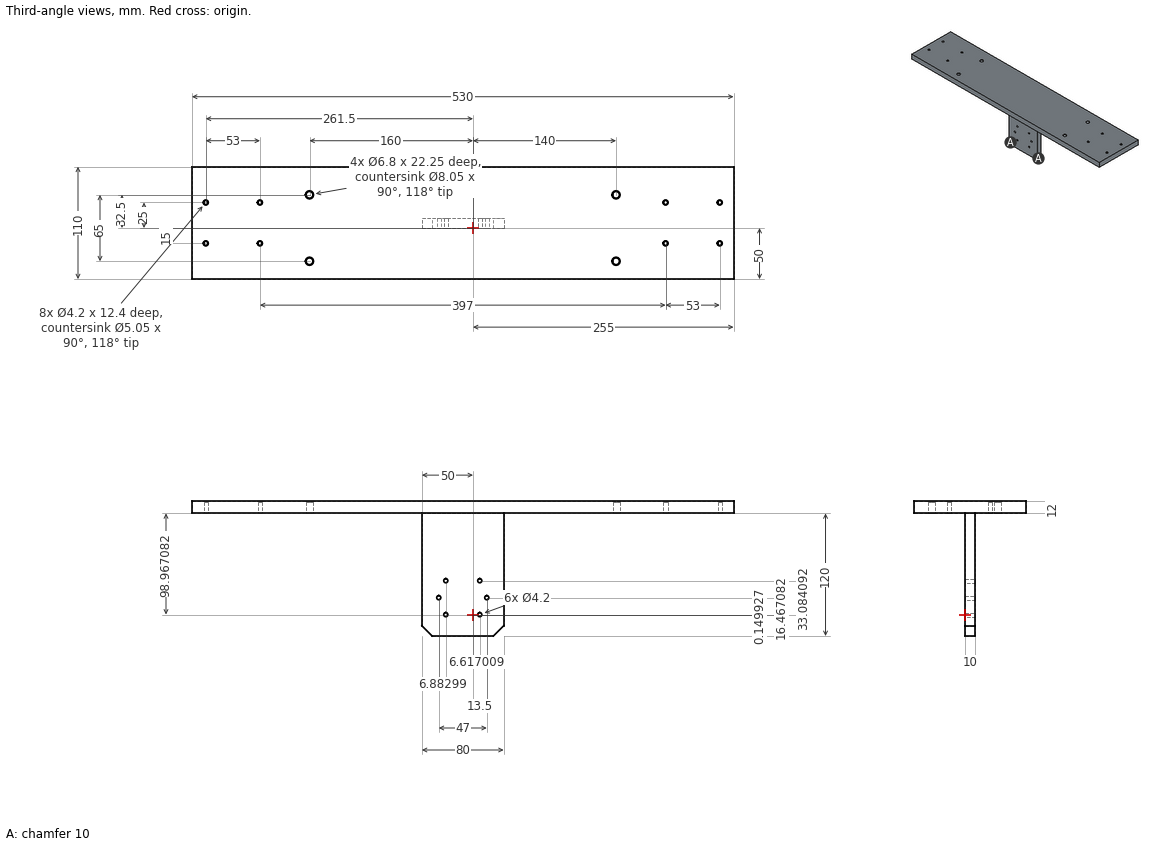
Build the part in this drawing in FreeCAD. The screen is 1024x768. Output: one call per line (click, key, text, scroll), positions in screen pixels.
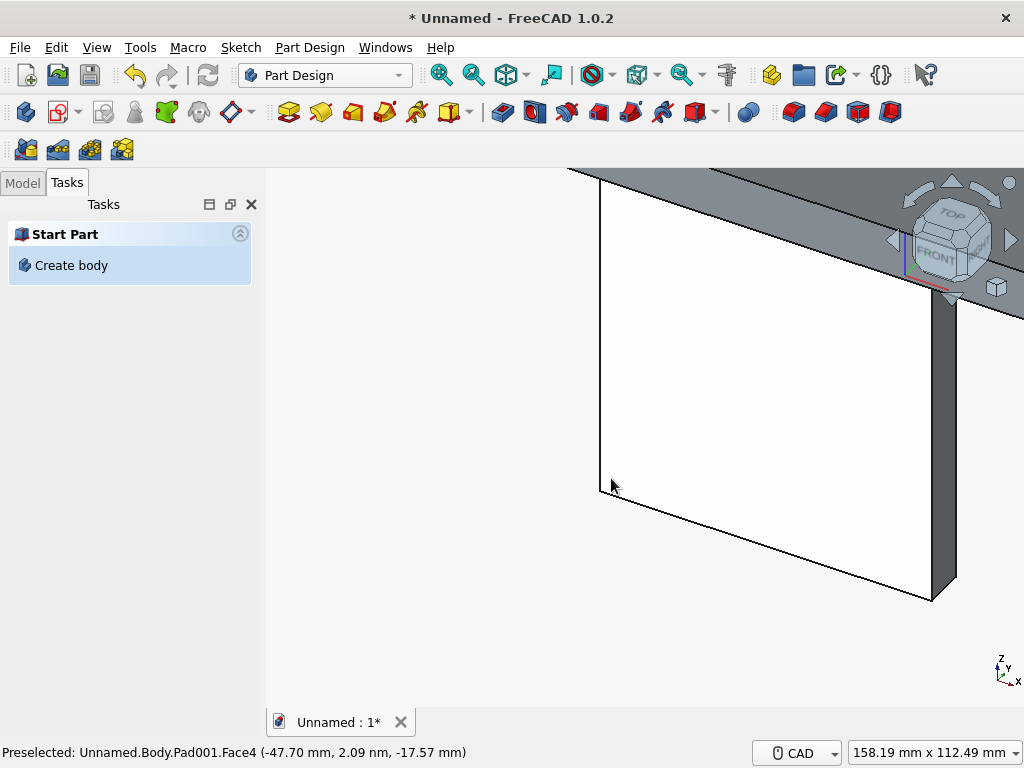
click(442, 76)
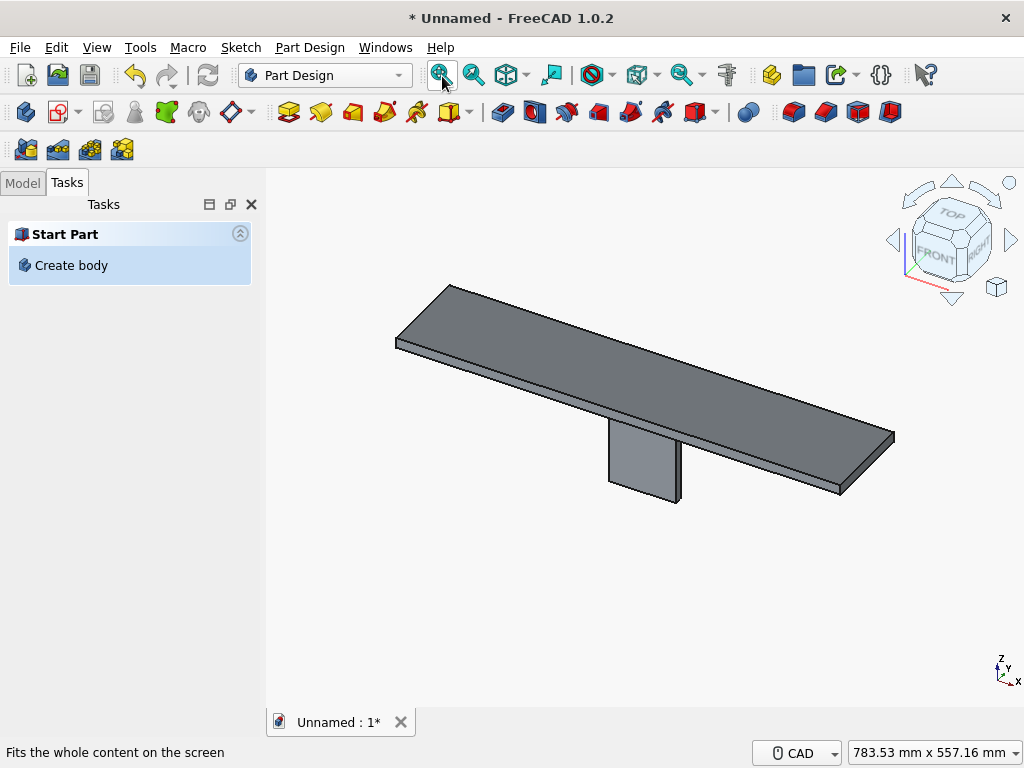
key(0)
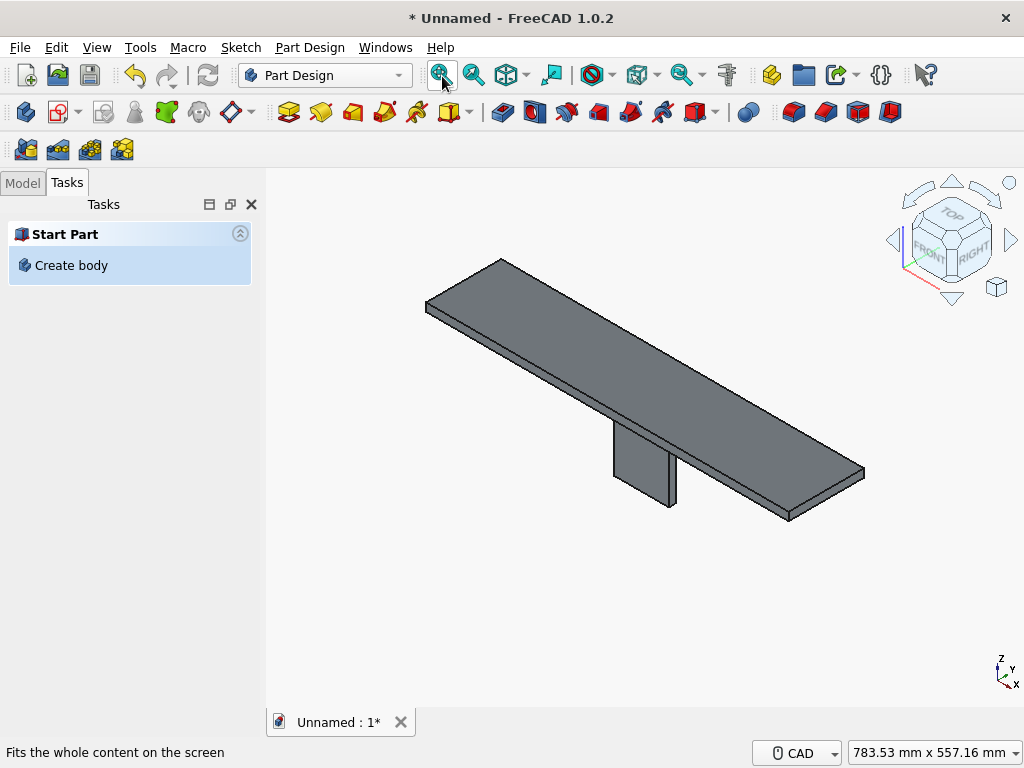
scroll(618, 473, up, 8)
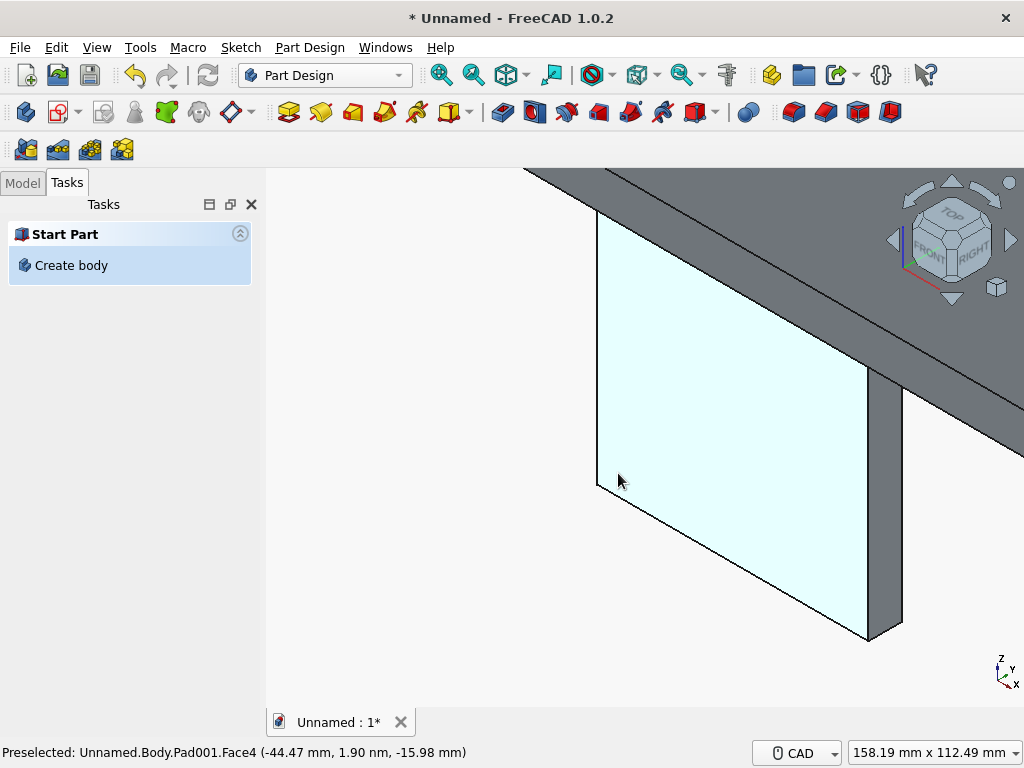
key(v)
key(f)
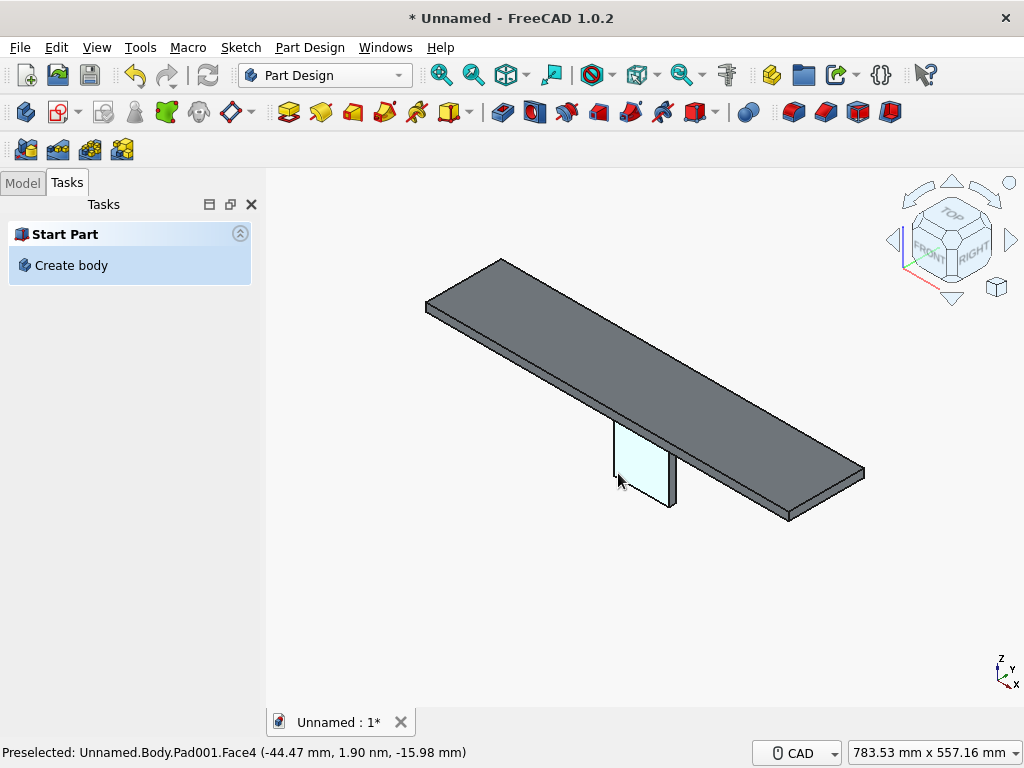
key(2)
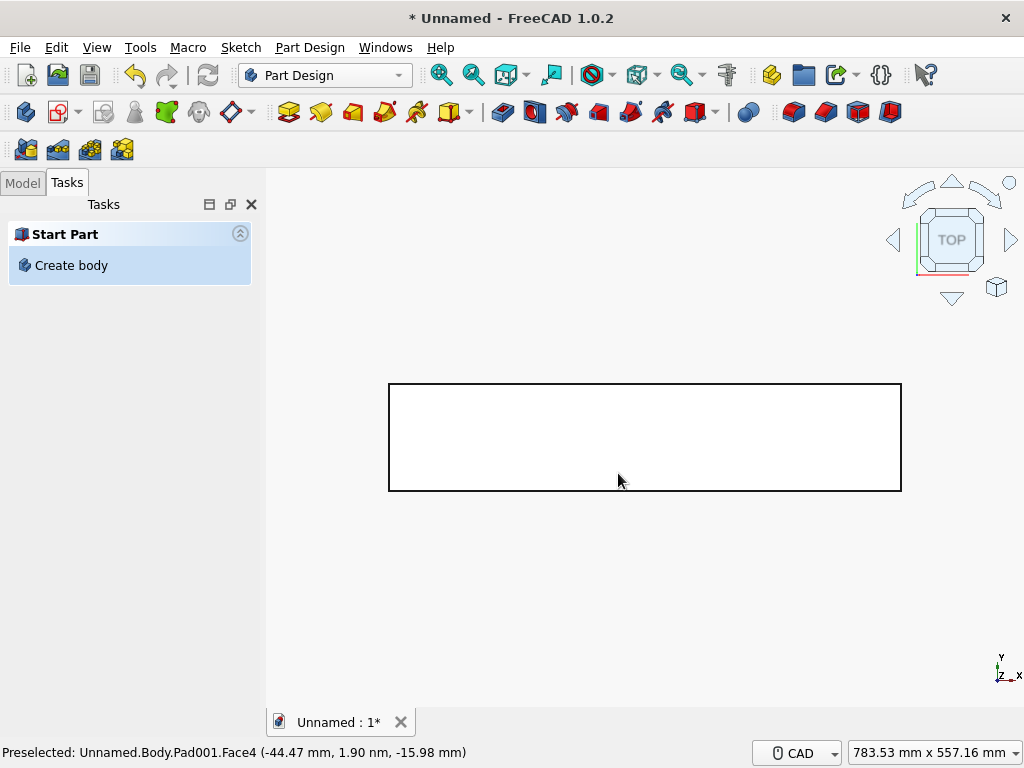
scroll(606, 436, up, 8)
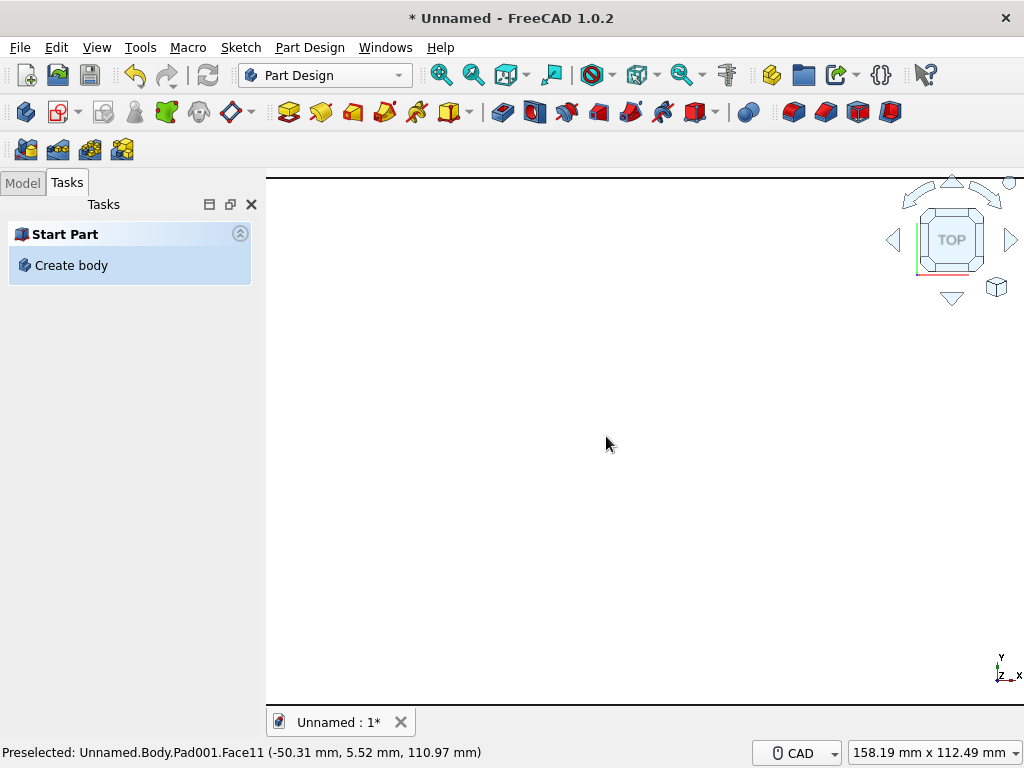
click(442, 76)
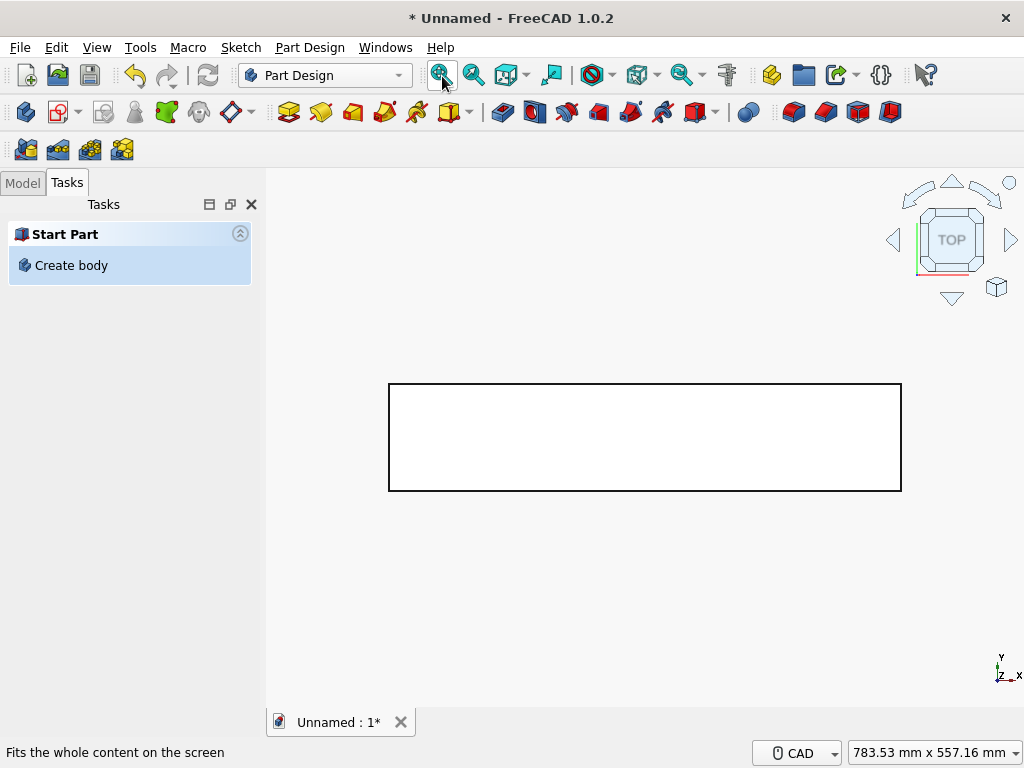
key(1)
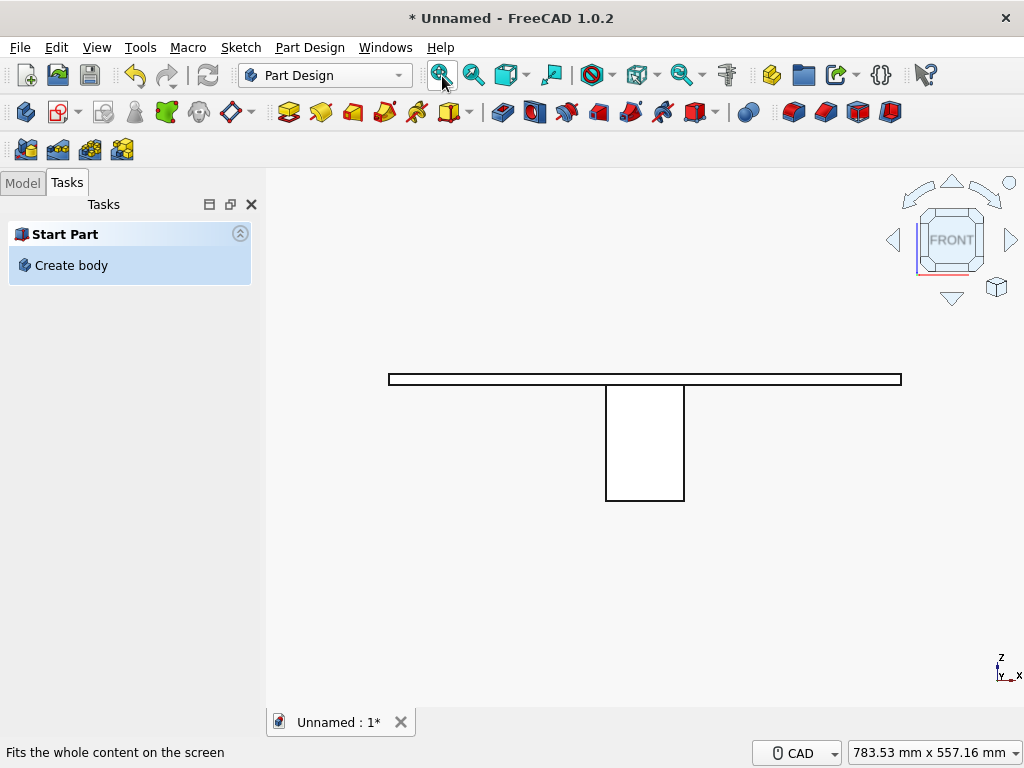
scroll(606, 500, up, 8)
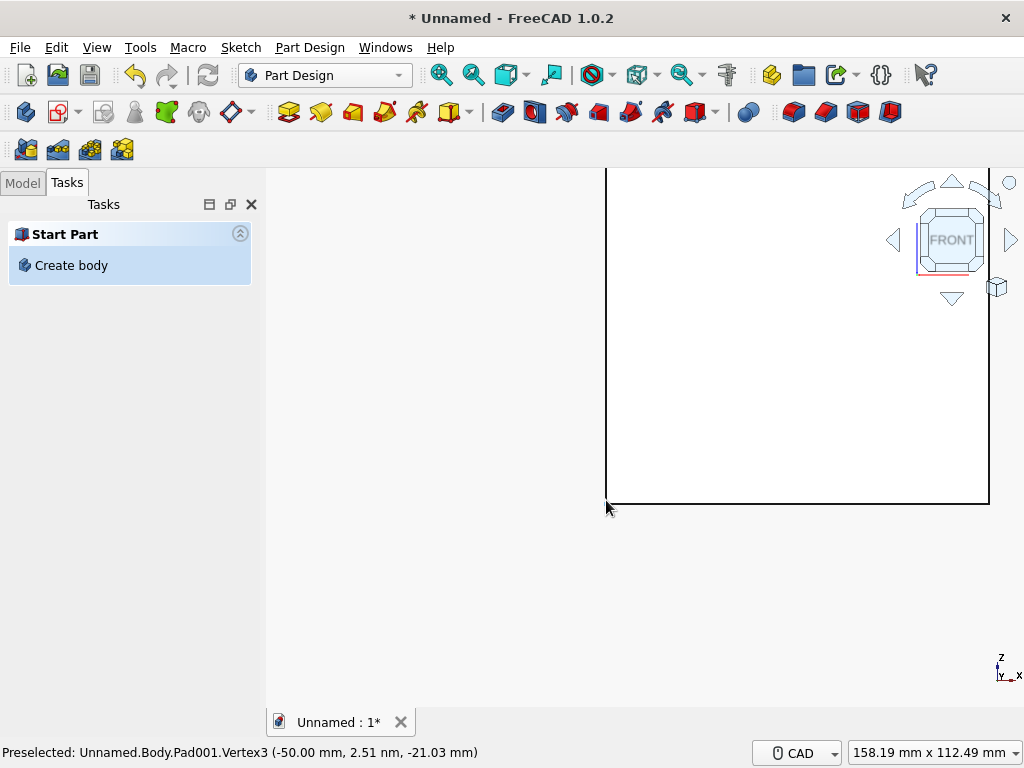
key(v)
key(f)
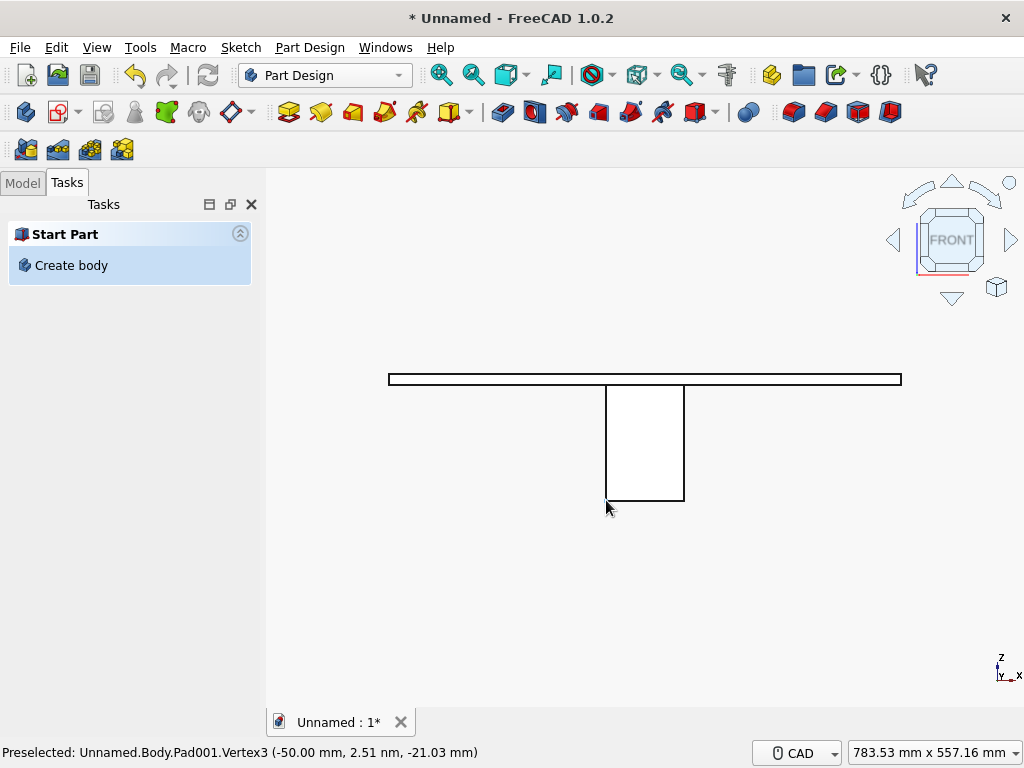
key(3)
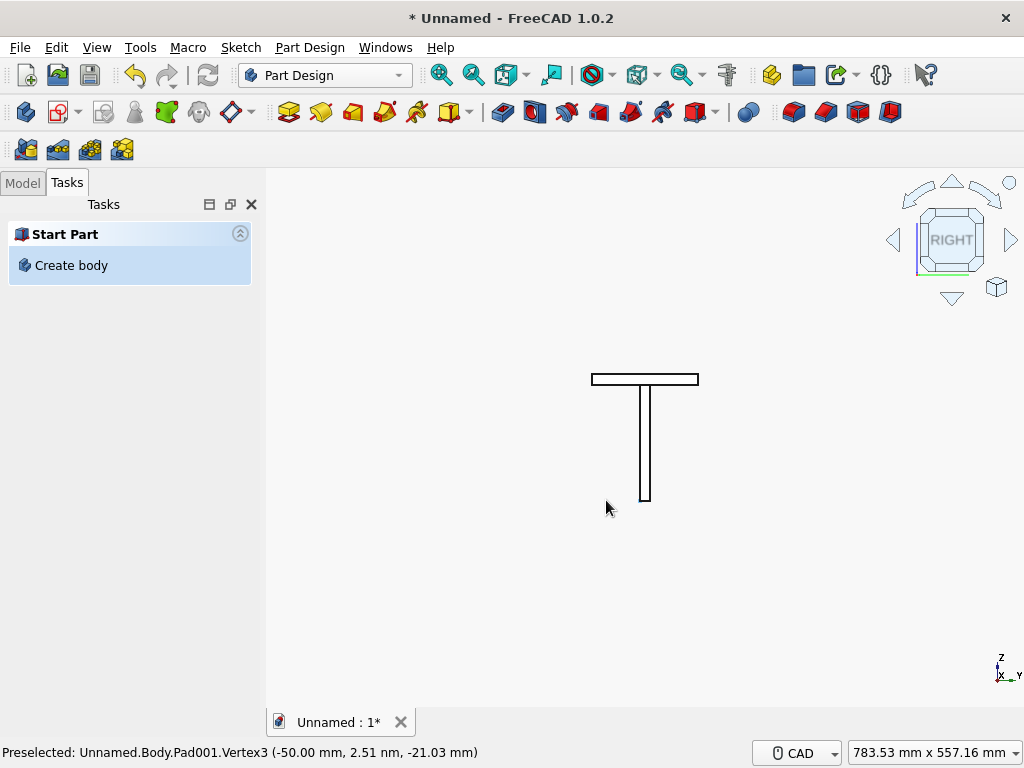
click(442, 76)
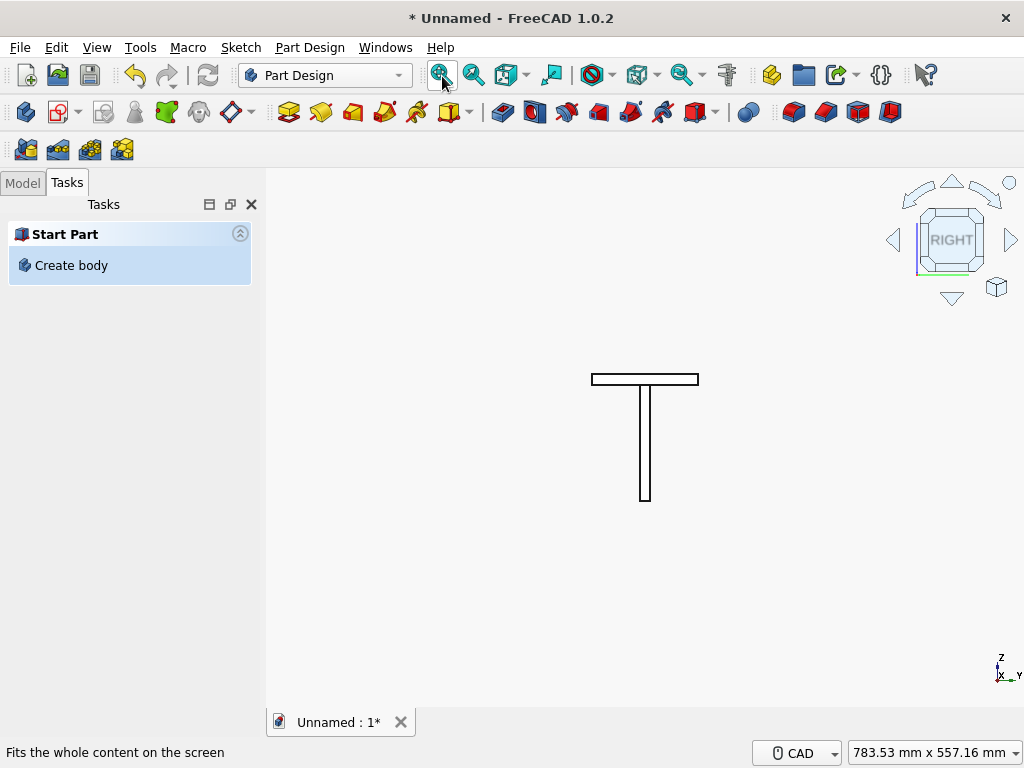
scroll(645, 500, up, 8)